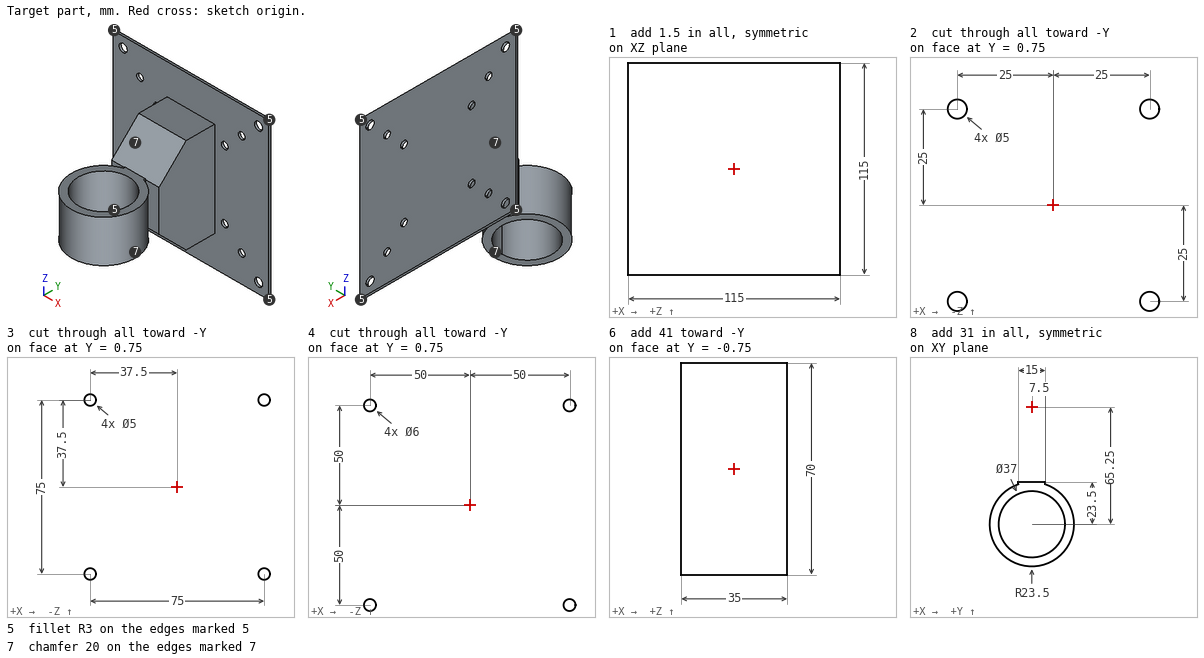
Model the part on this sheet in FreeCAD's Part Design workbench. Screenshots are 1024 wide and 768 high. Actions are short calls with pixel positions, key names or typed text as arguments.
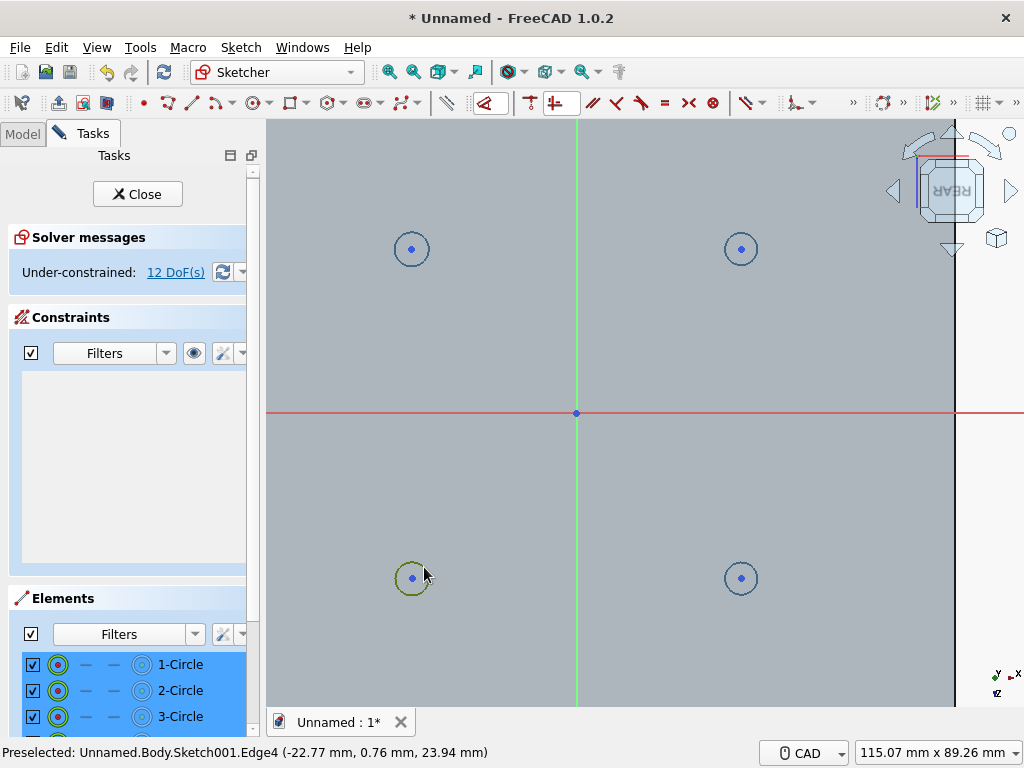
key(e)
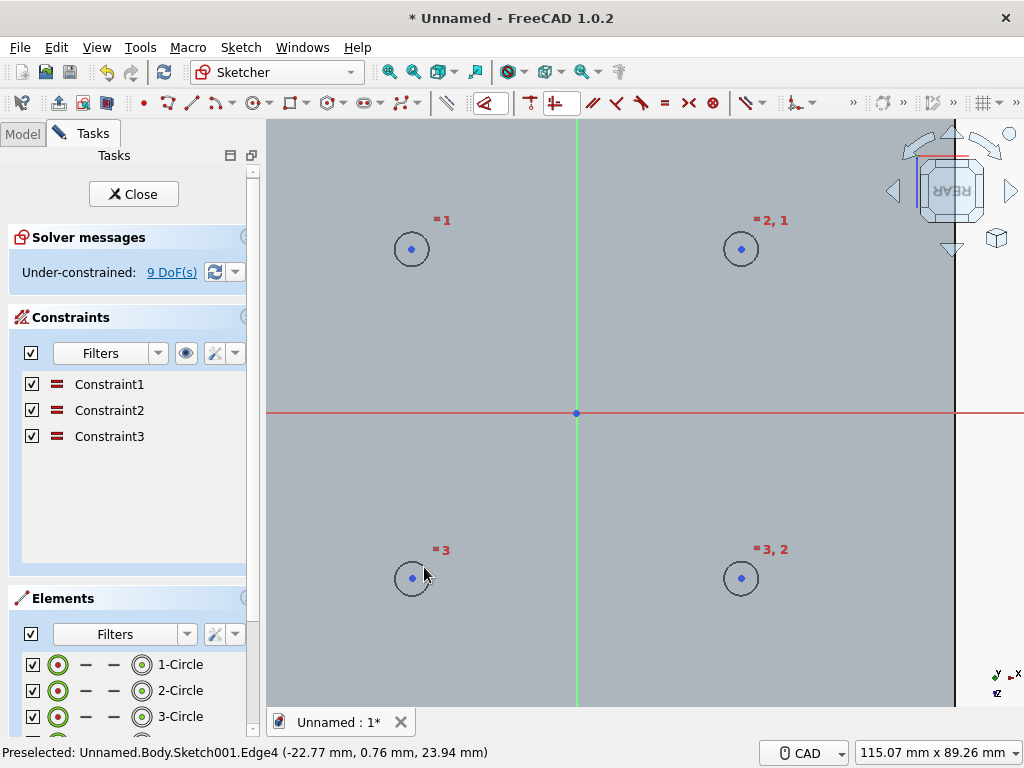
click(412, 249)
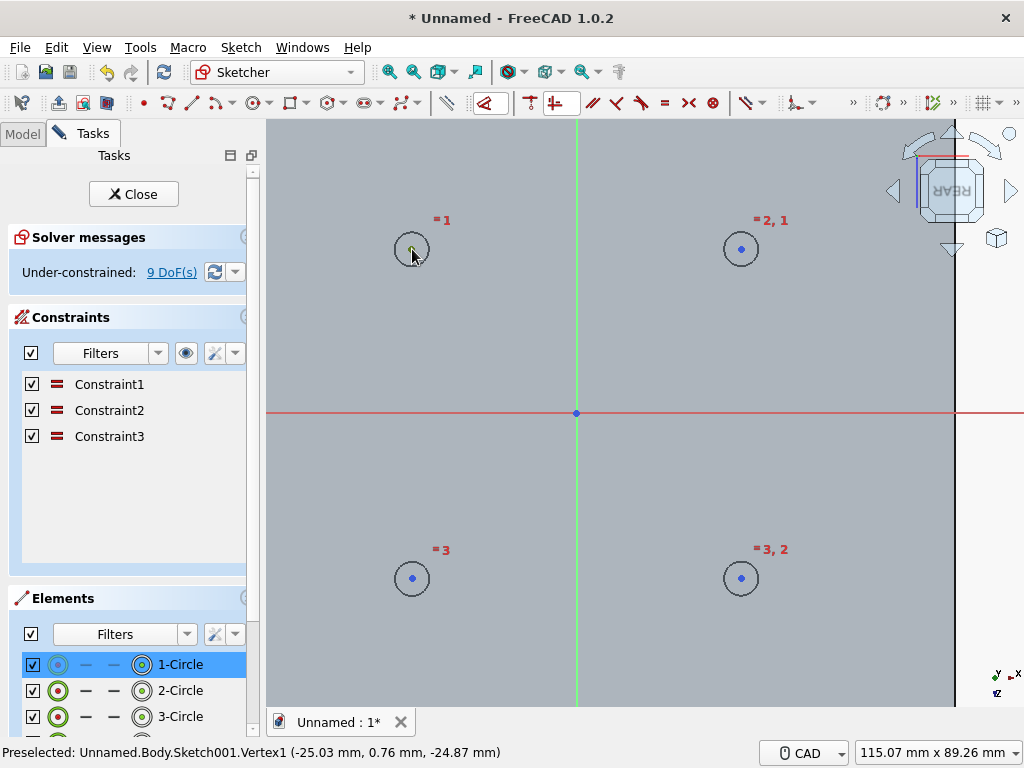
click(741, 249)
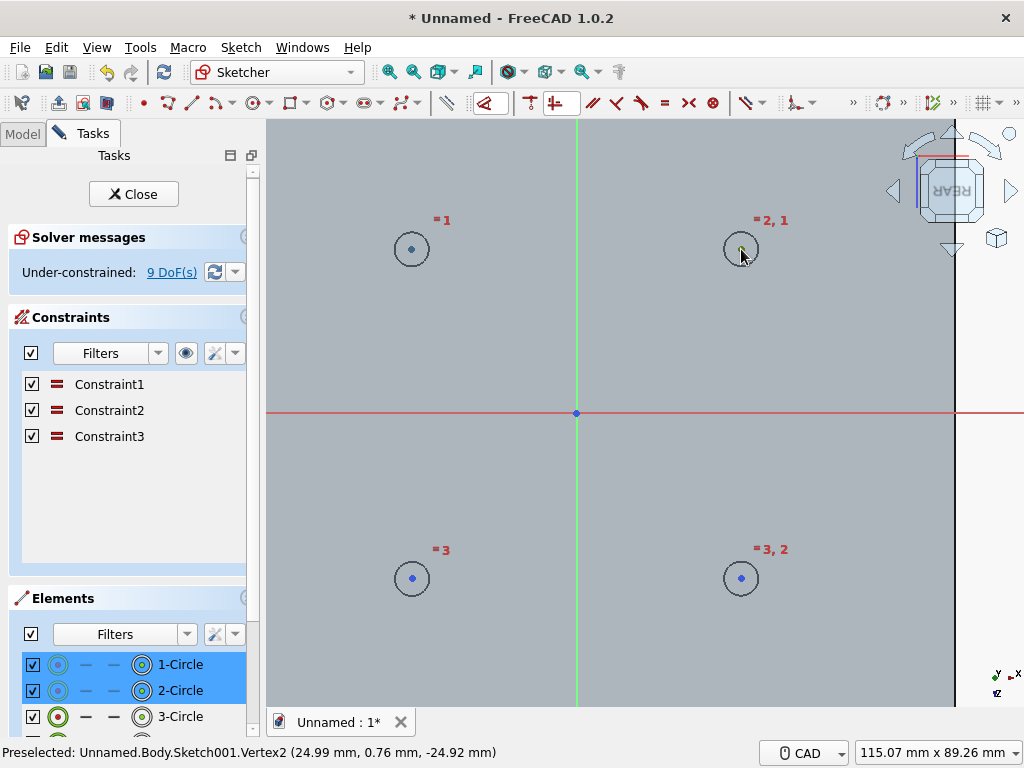
key(h)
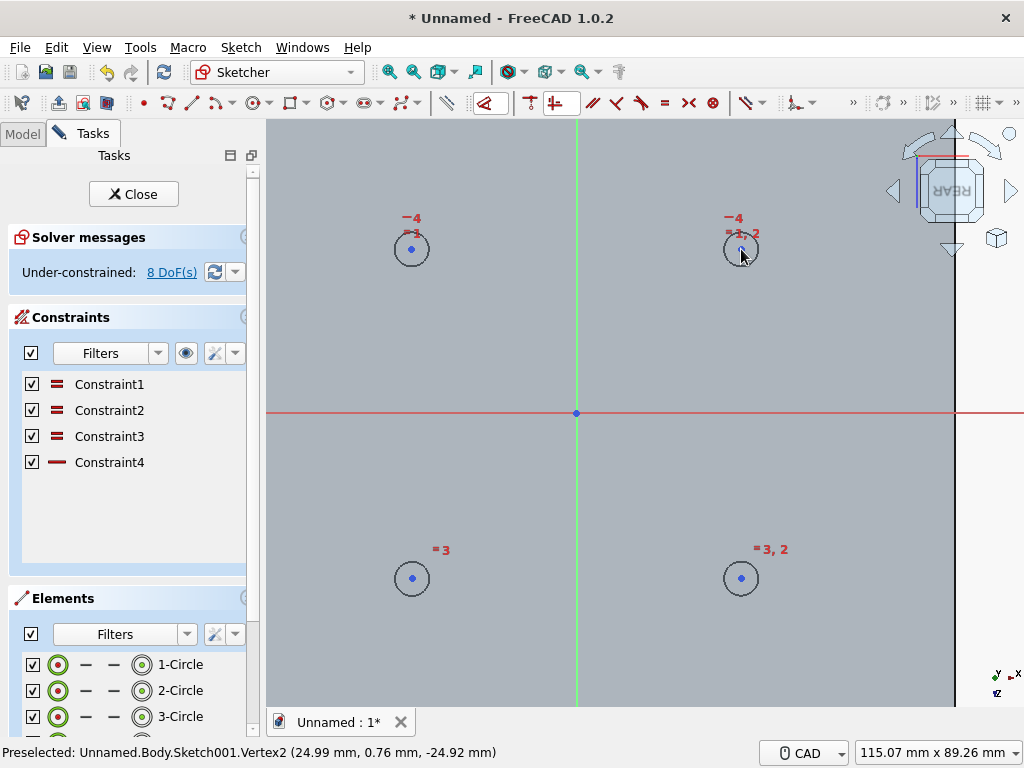
click(741, 249)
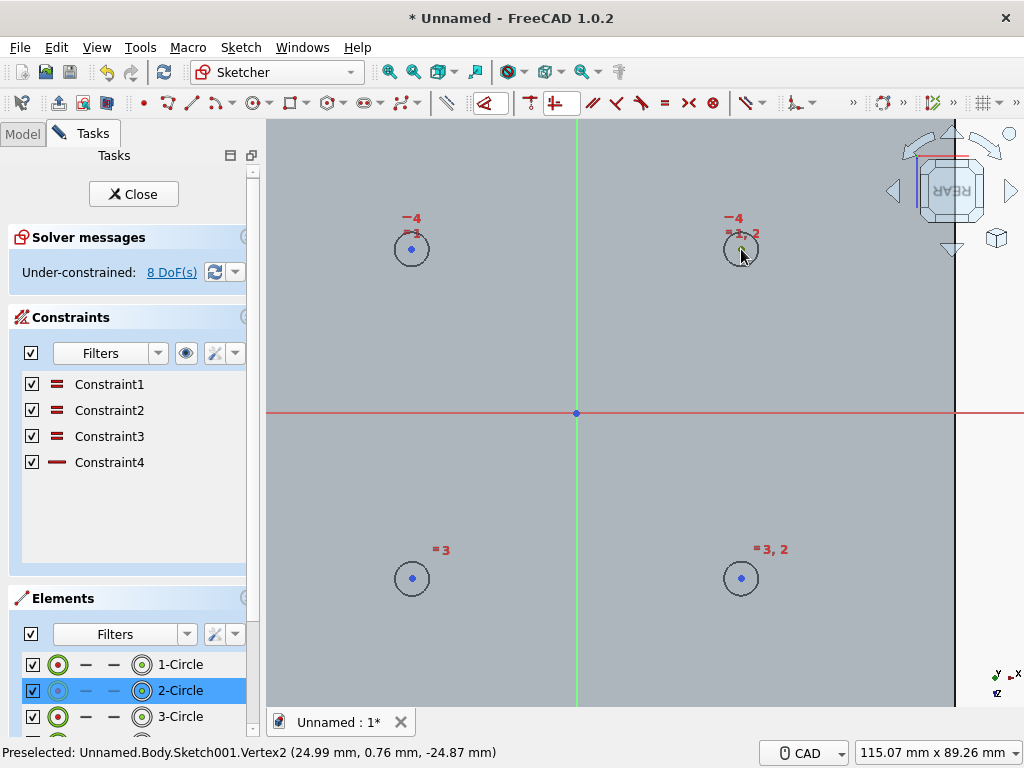
click(741, 579)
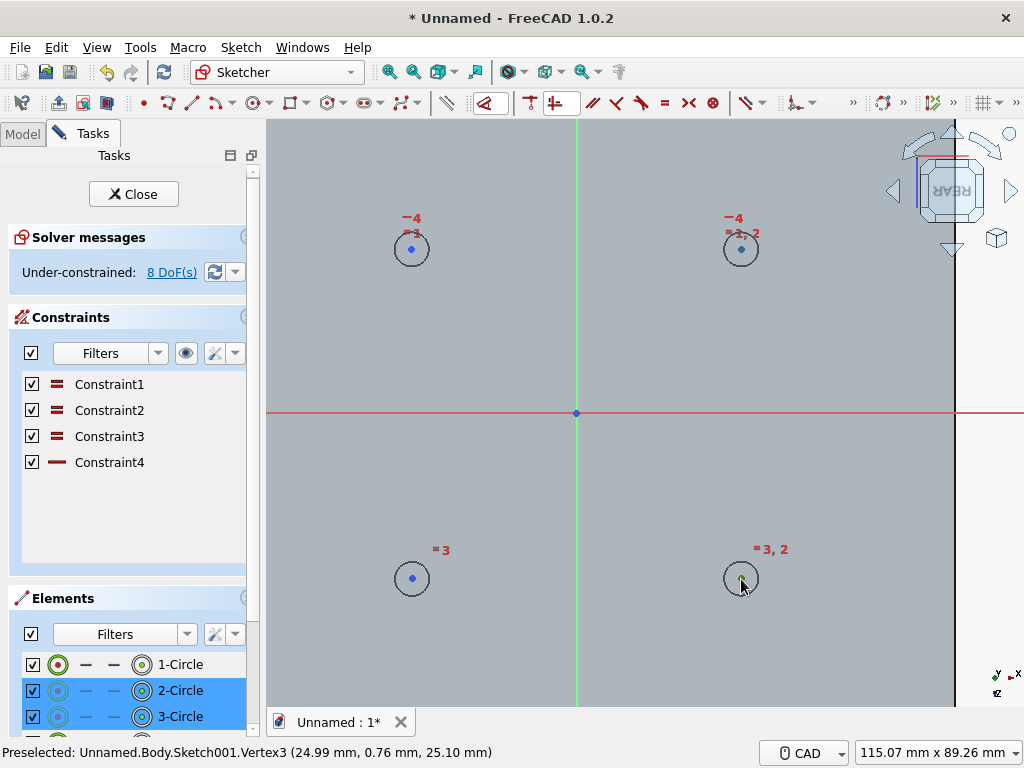
key(v)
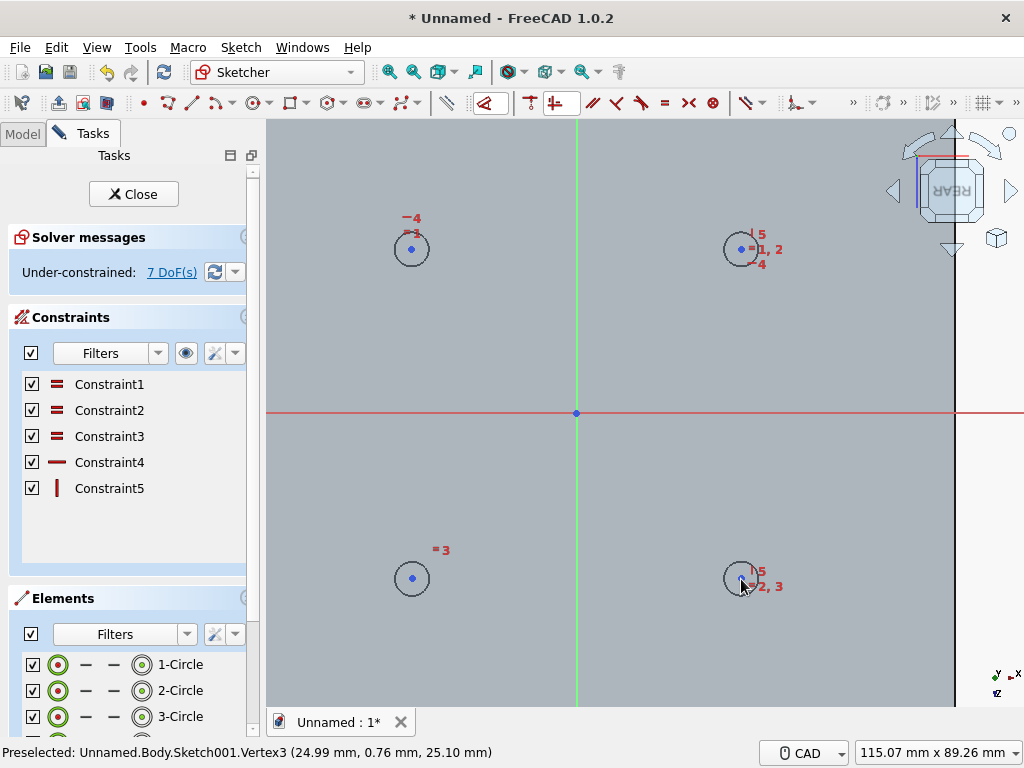
click(412, 249)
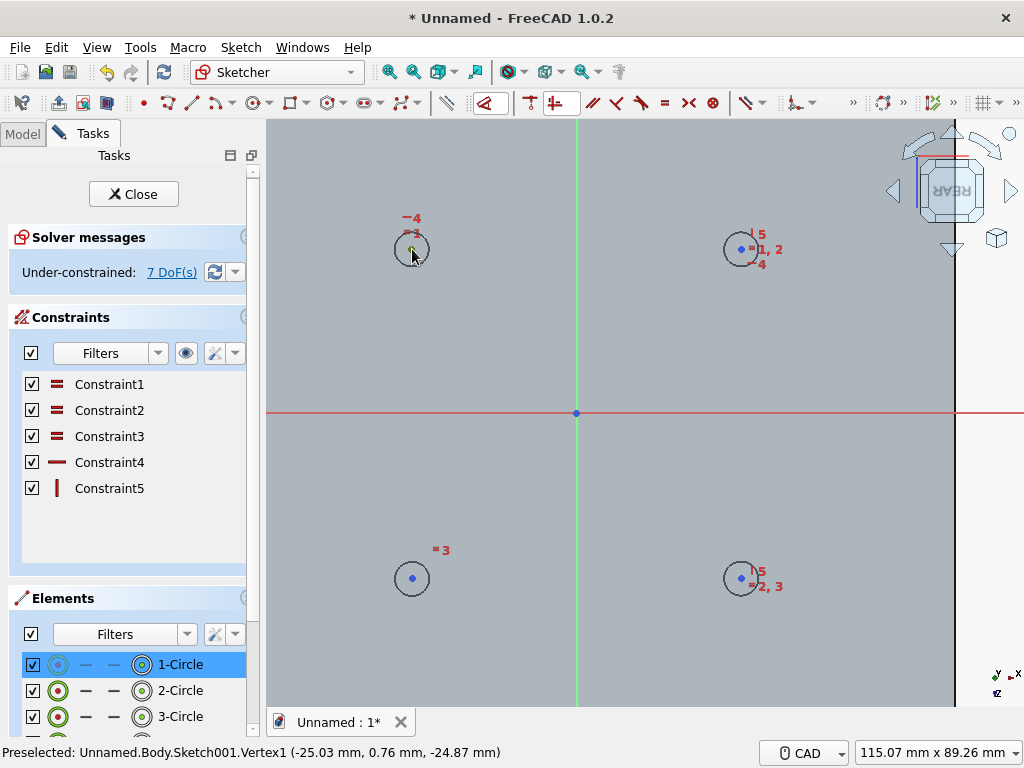
click(412, 579)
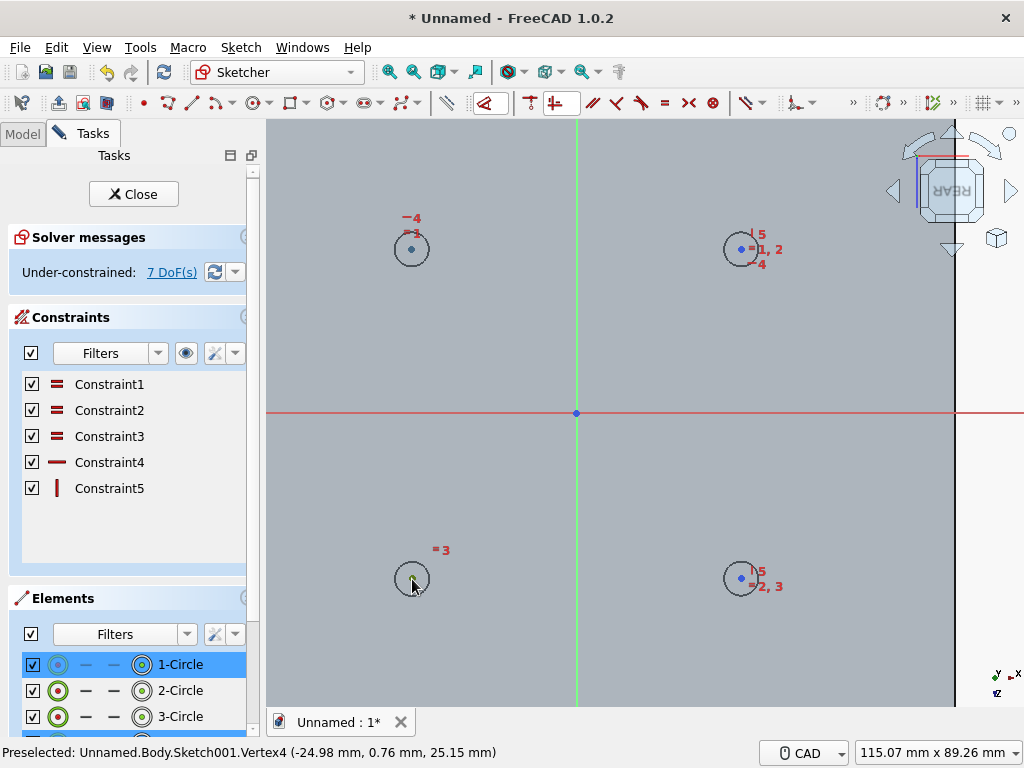
key(v)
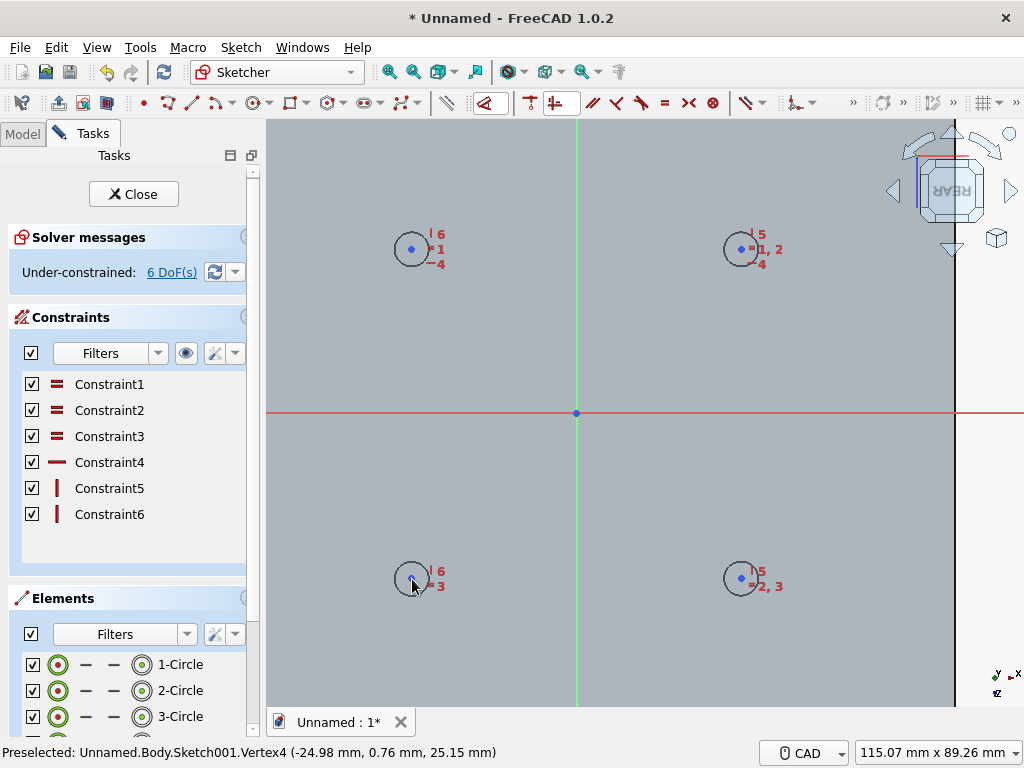
click(741, 579)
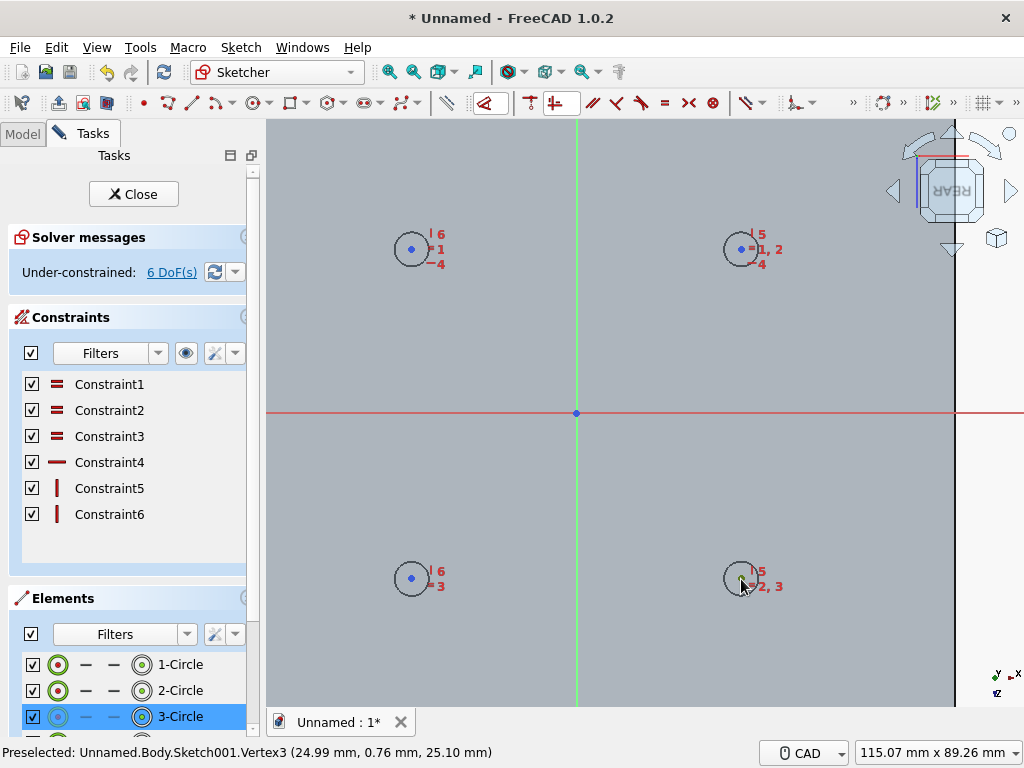
click(412, 579)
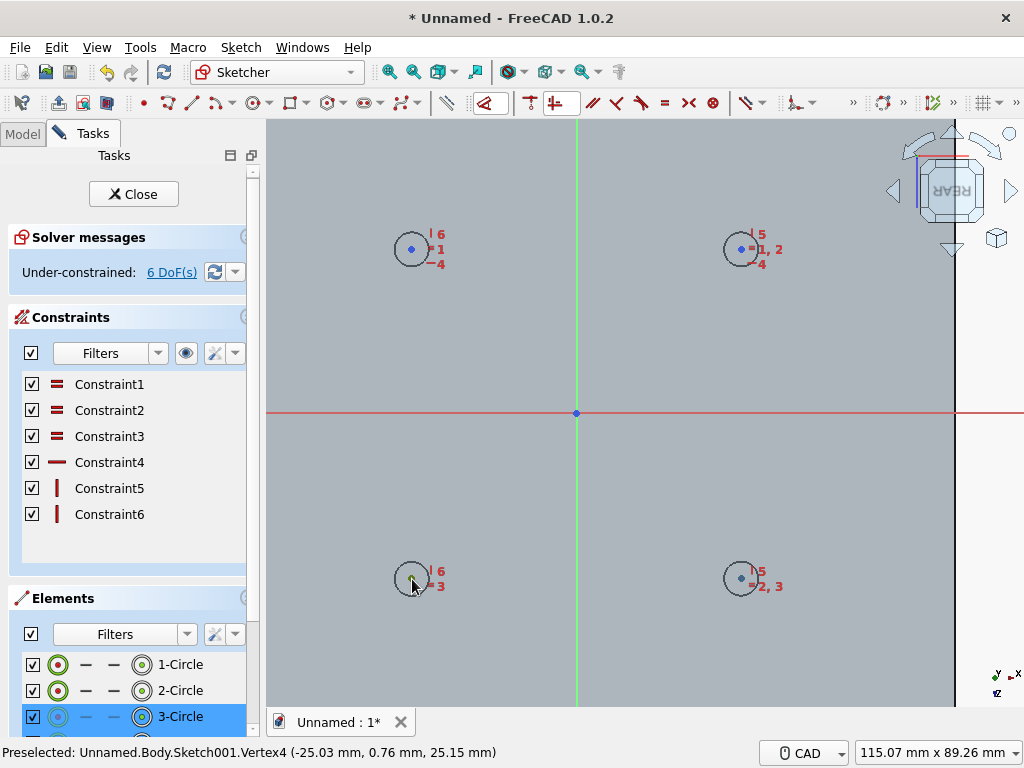
key(h)